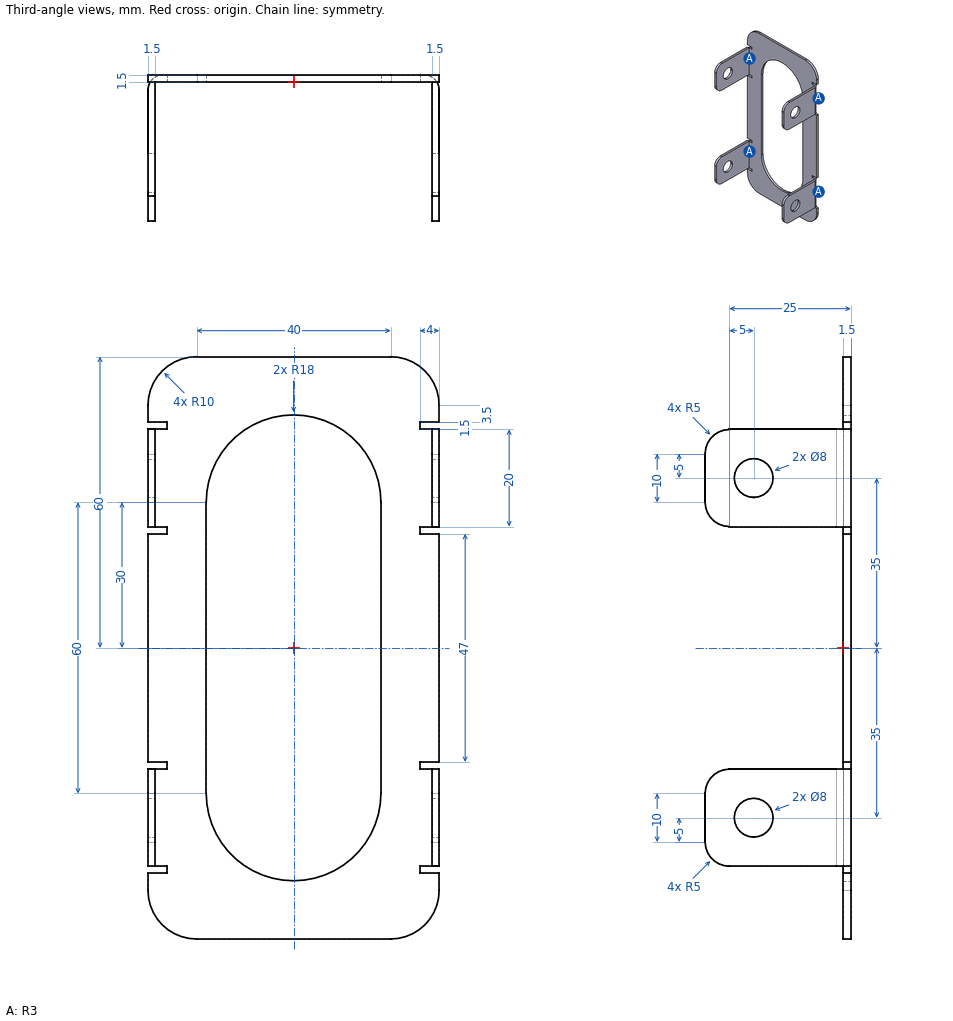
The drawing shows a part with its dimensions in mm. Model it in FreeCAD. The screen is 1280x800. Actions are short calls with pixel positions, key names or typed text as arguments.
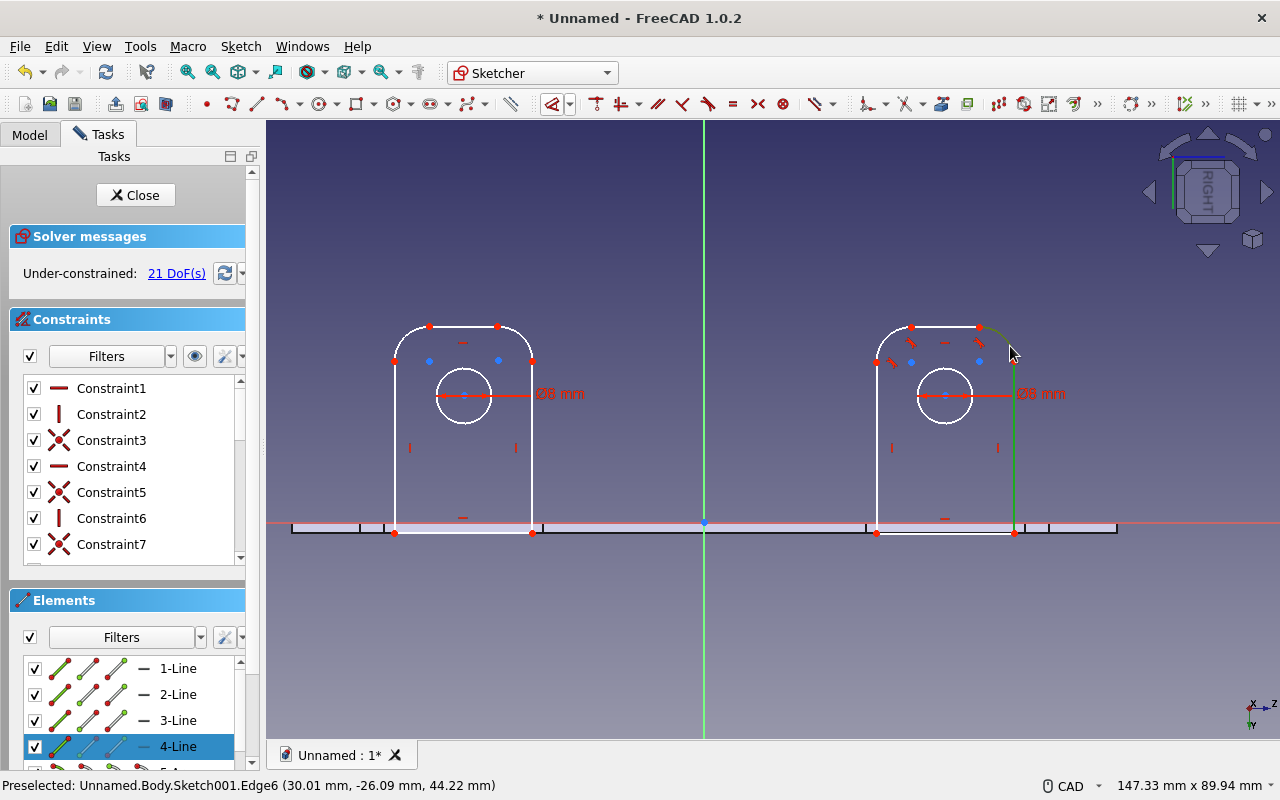
key(t)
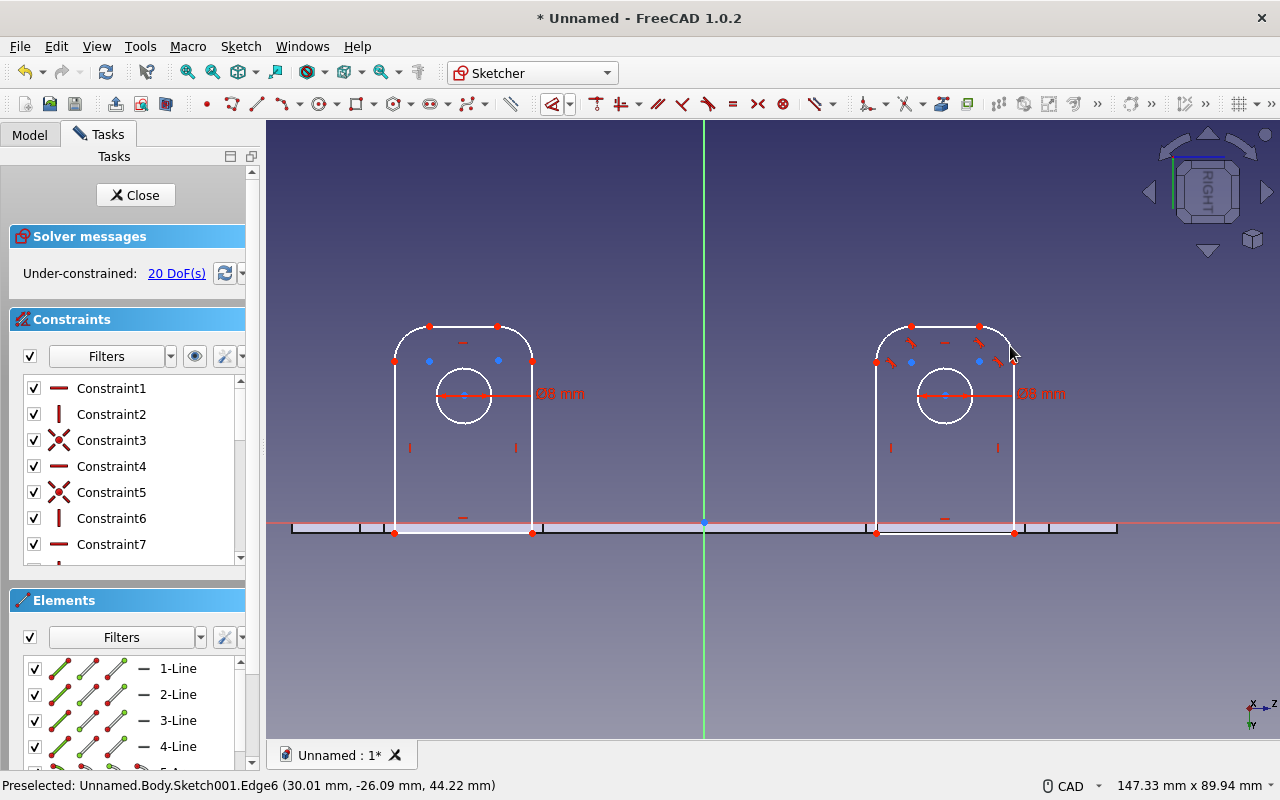
click(477, 327)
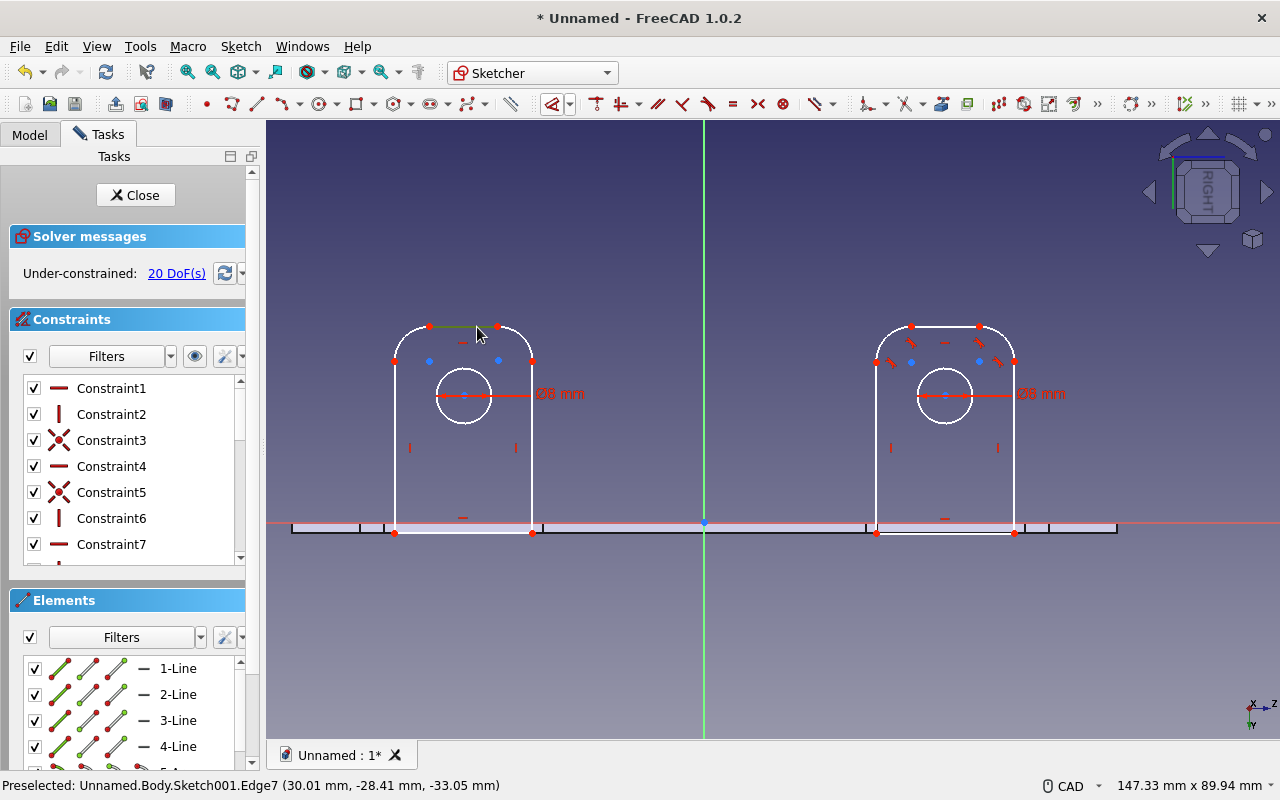
click(414, 331)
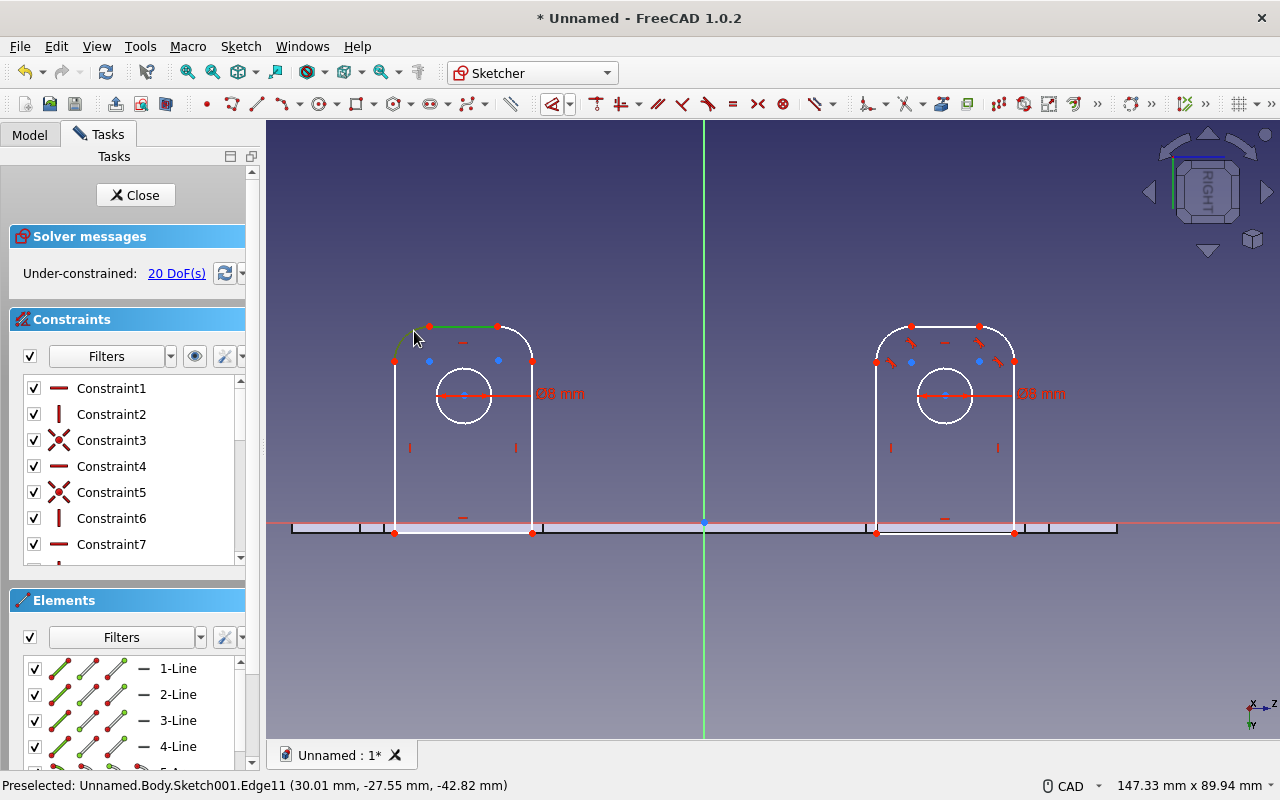
click(708, 104)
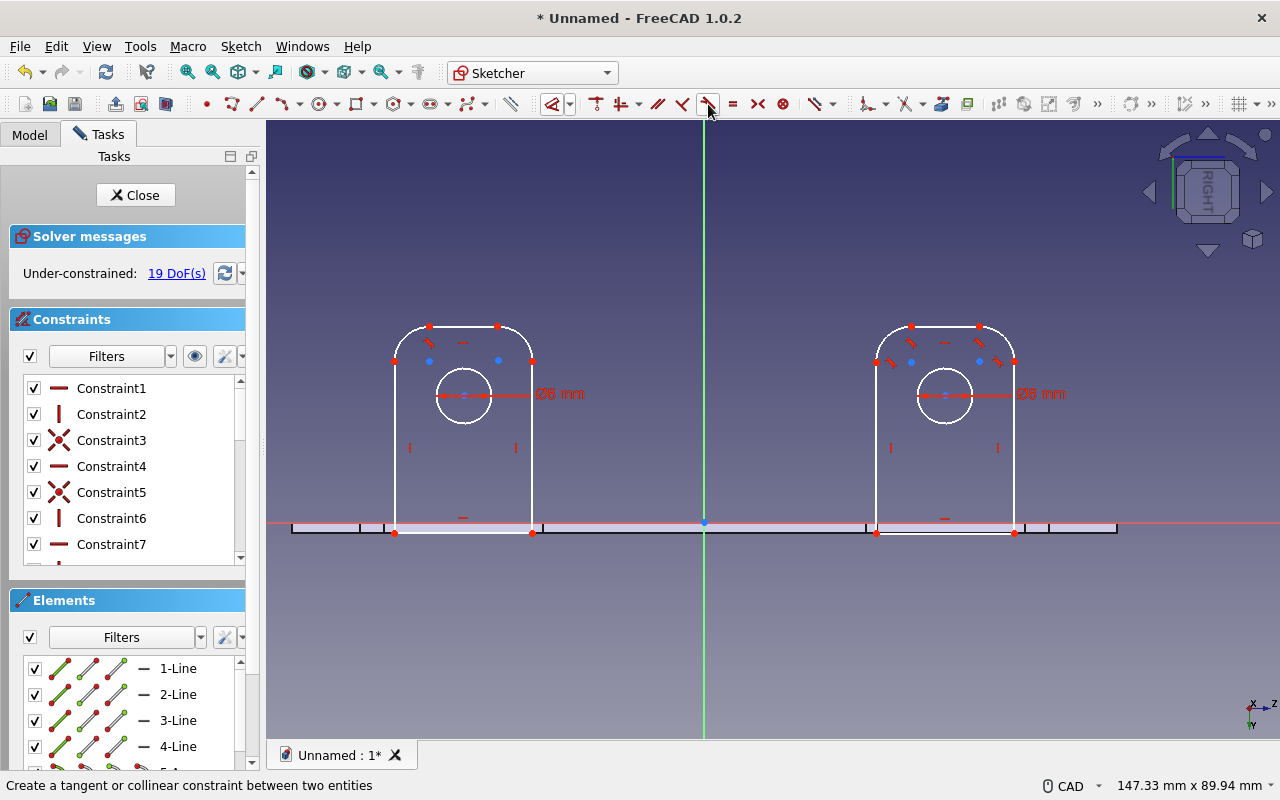
click(477, 327)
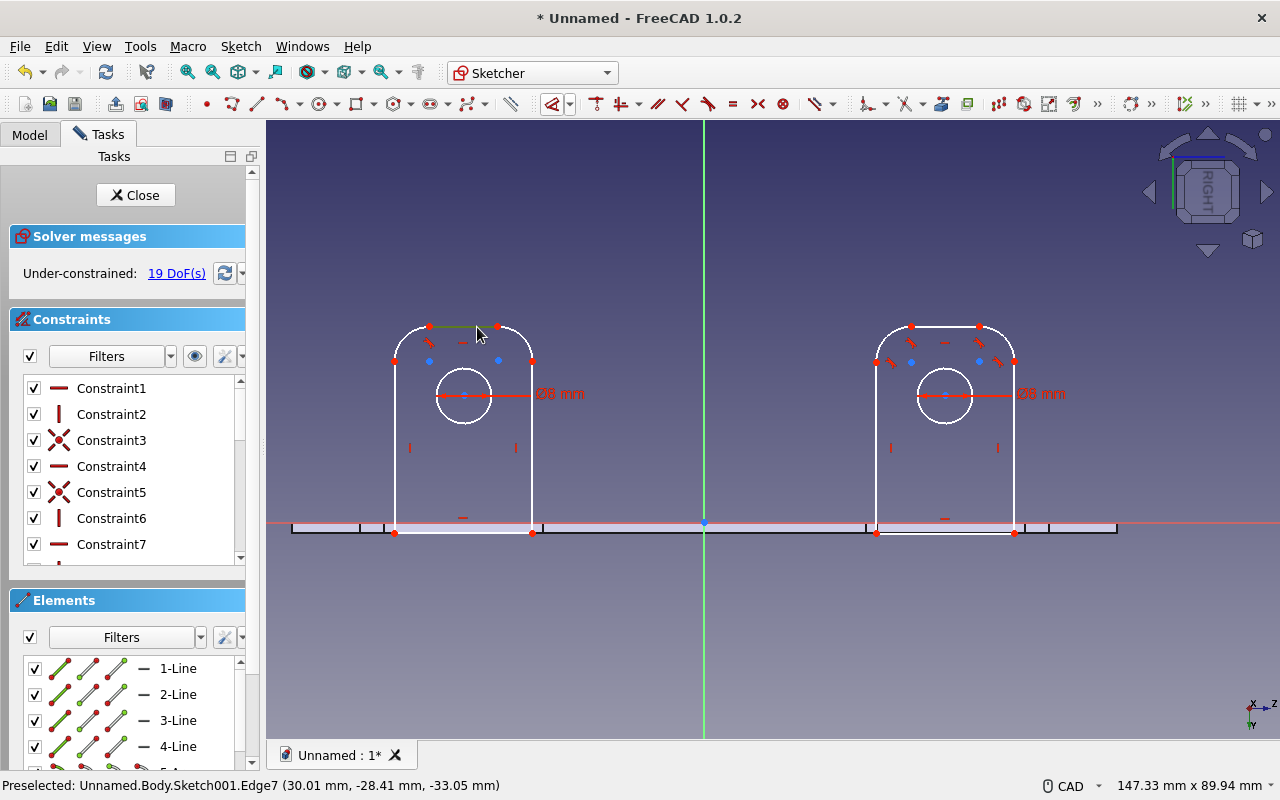
click(529, 346)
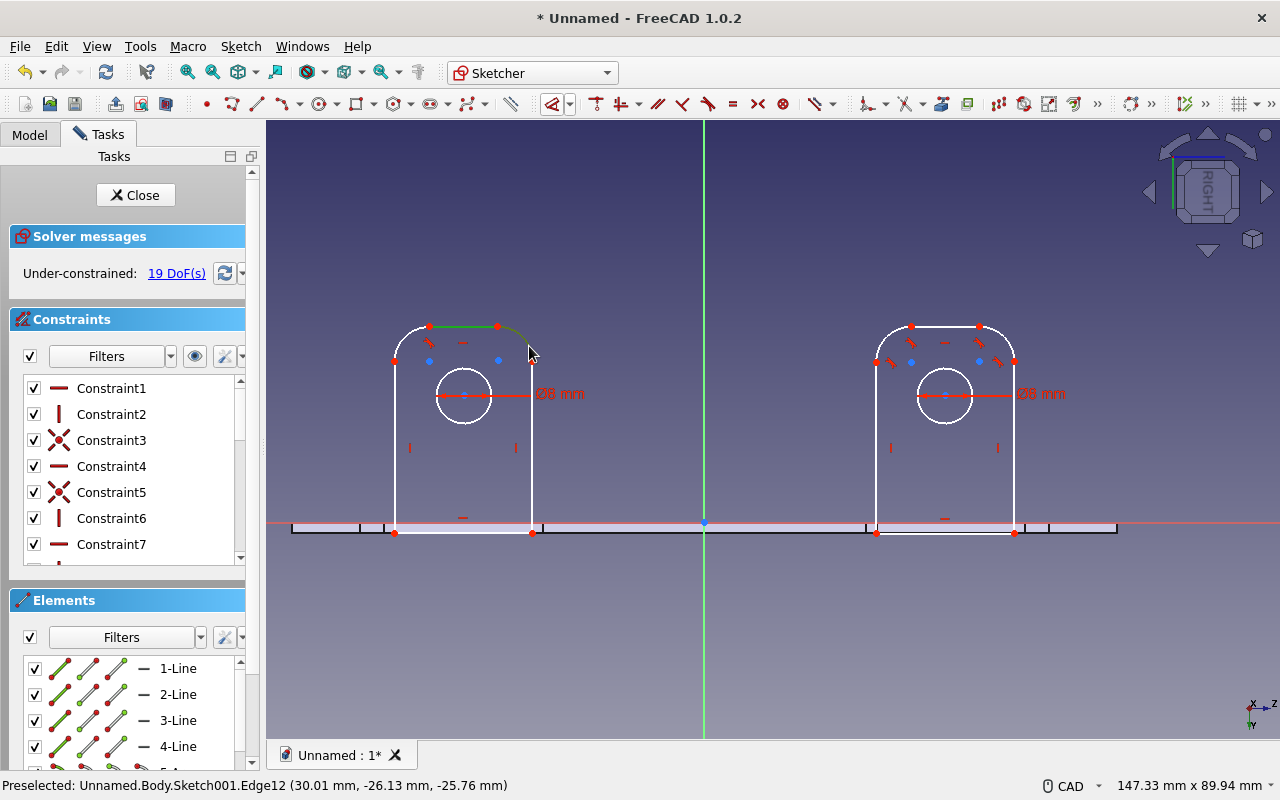
click(708, 104)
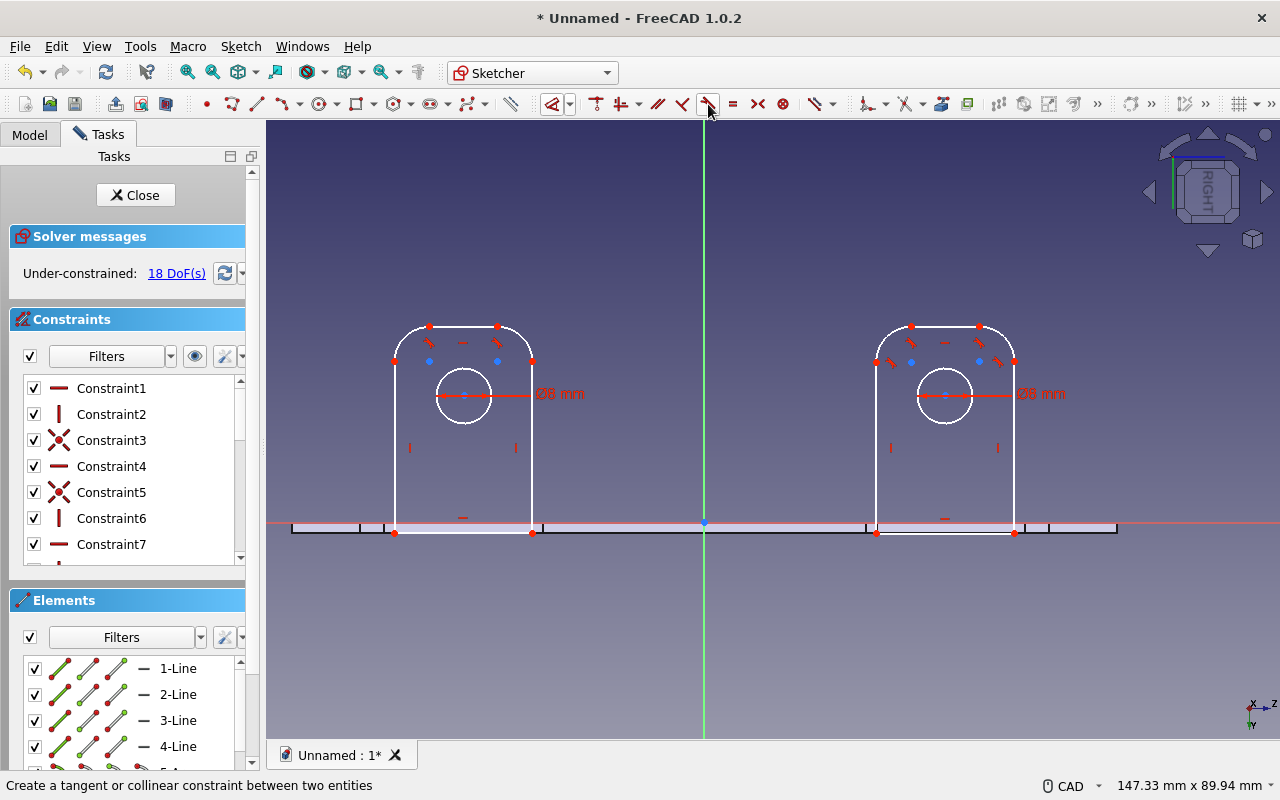
click(395, 413)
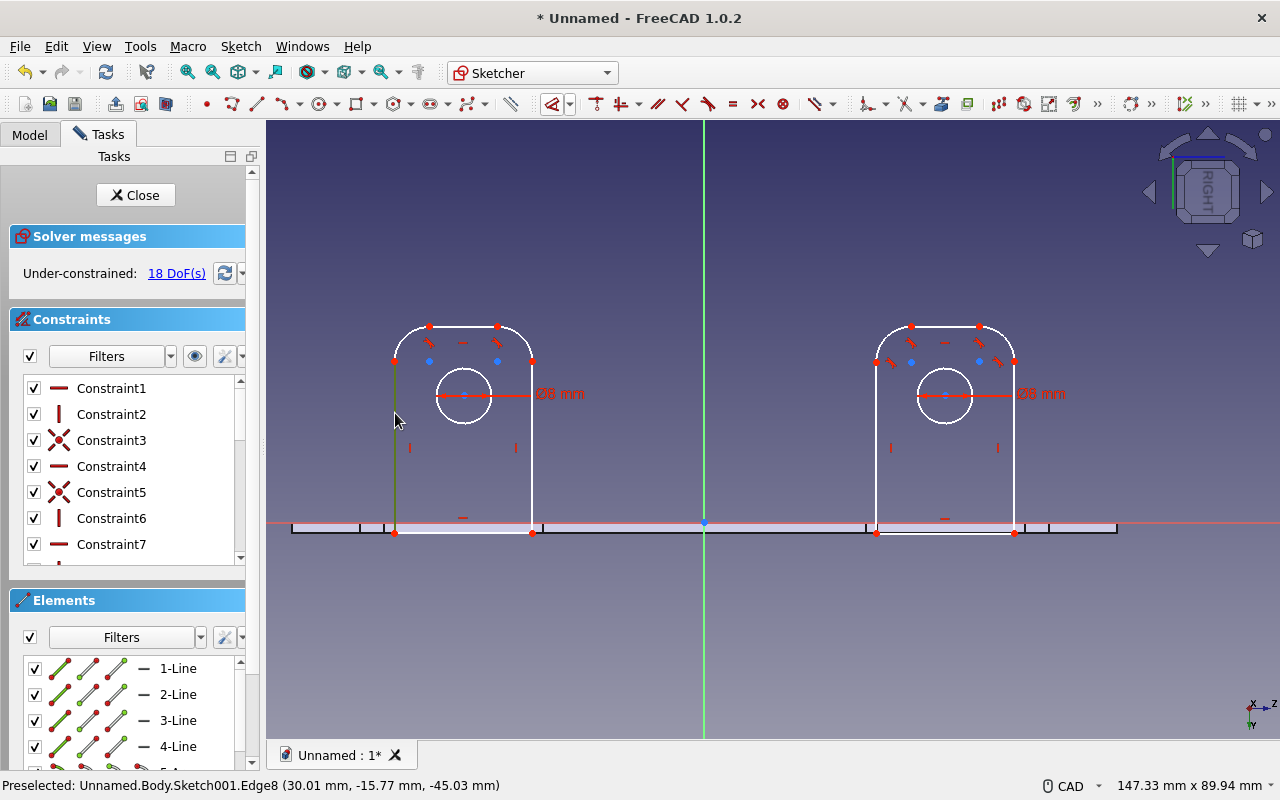
click(414, 331)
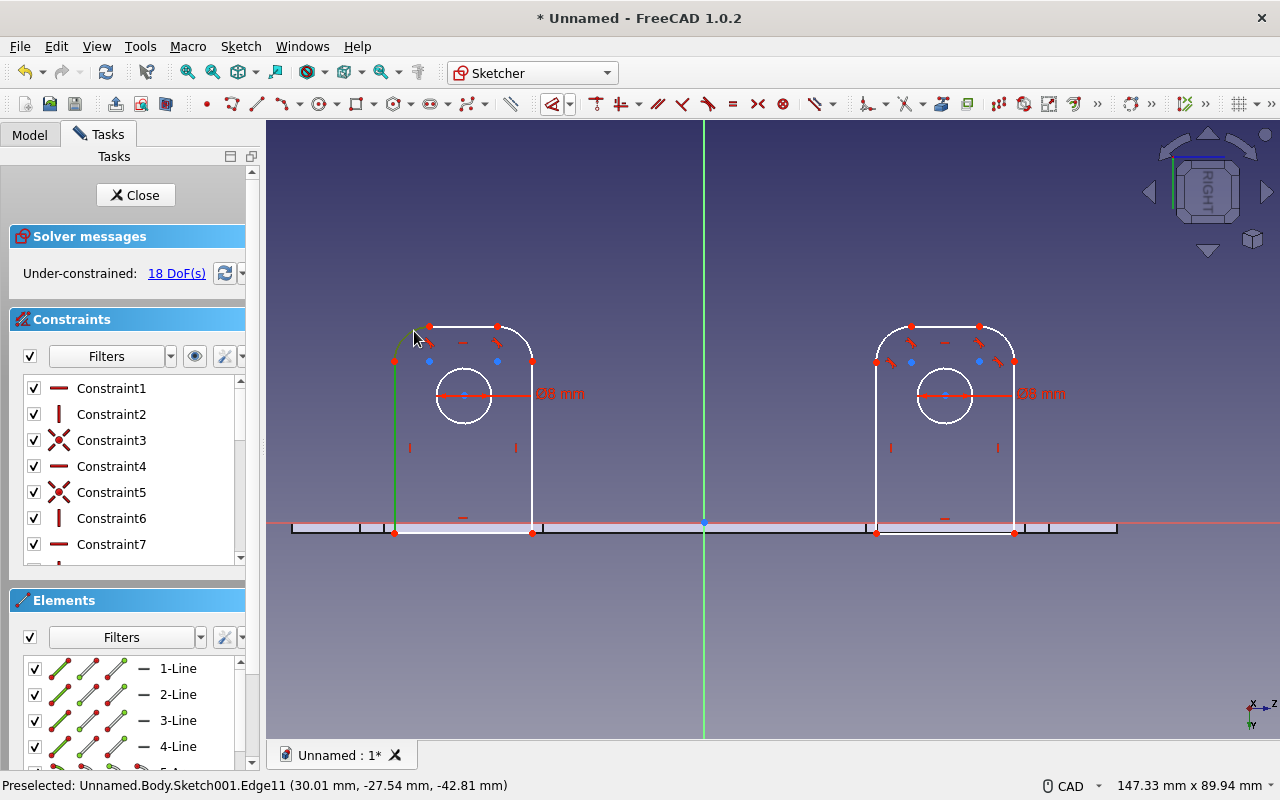
click(708, 104)